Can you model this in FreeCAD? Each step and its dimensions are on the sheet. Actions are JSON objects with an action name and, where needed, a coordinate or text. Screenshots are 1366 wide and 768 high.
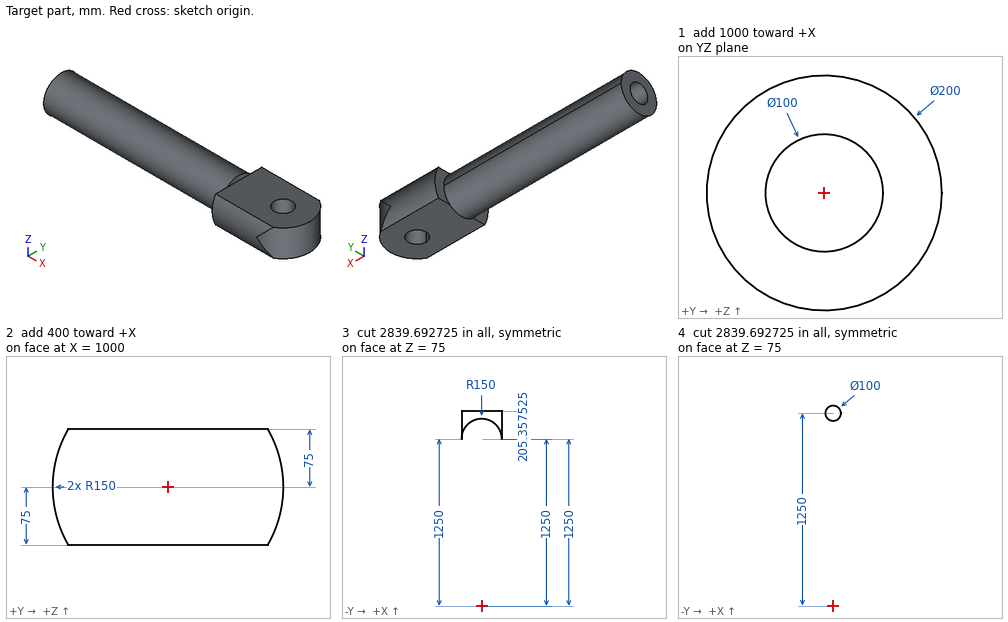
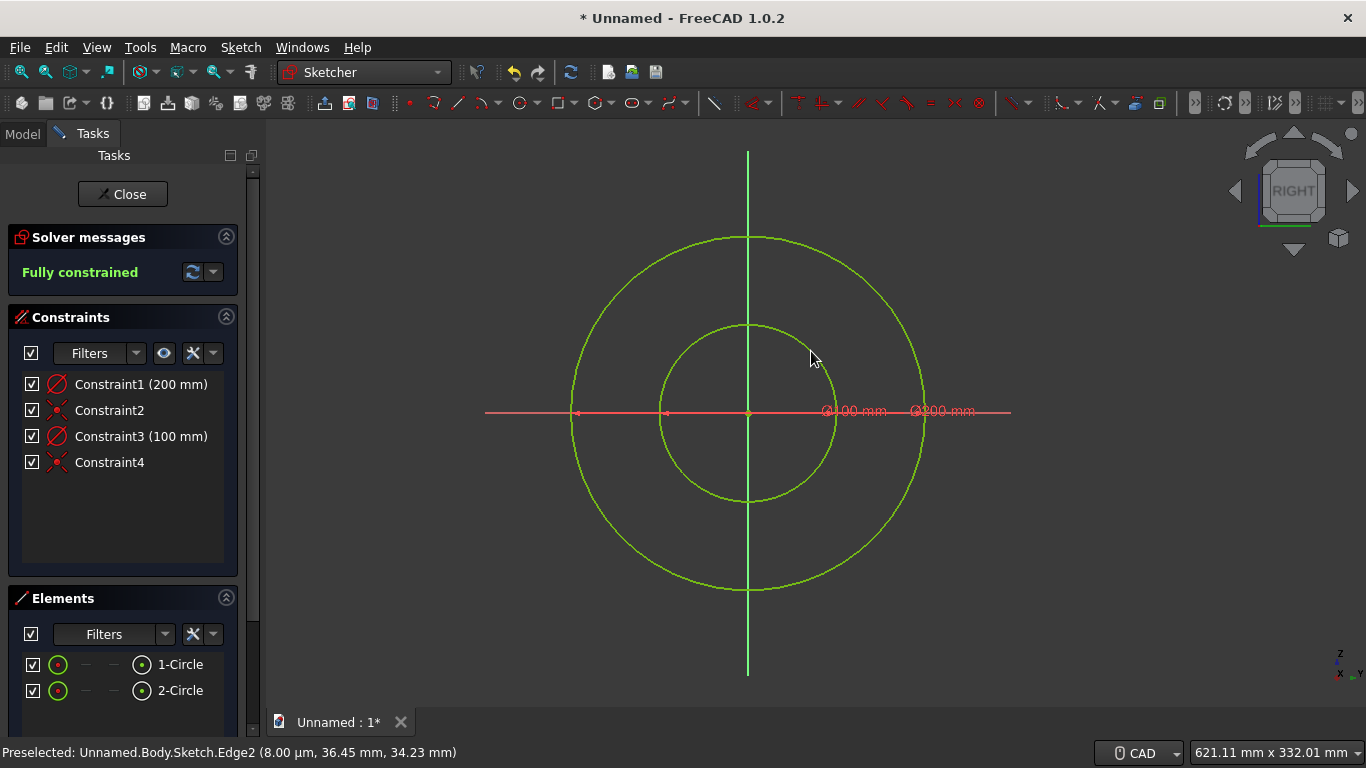
{"action": "left_click", "coordinate": [123, 194]}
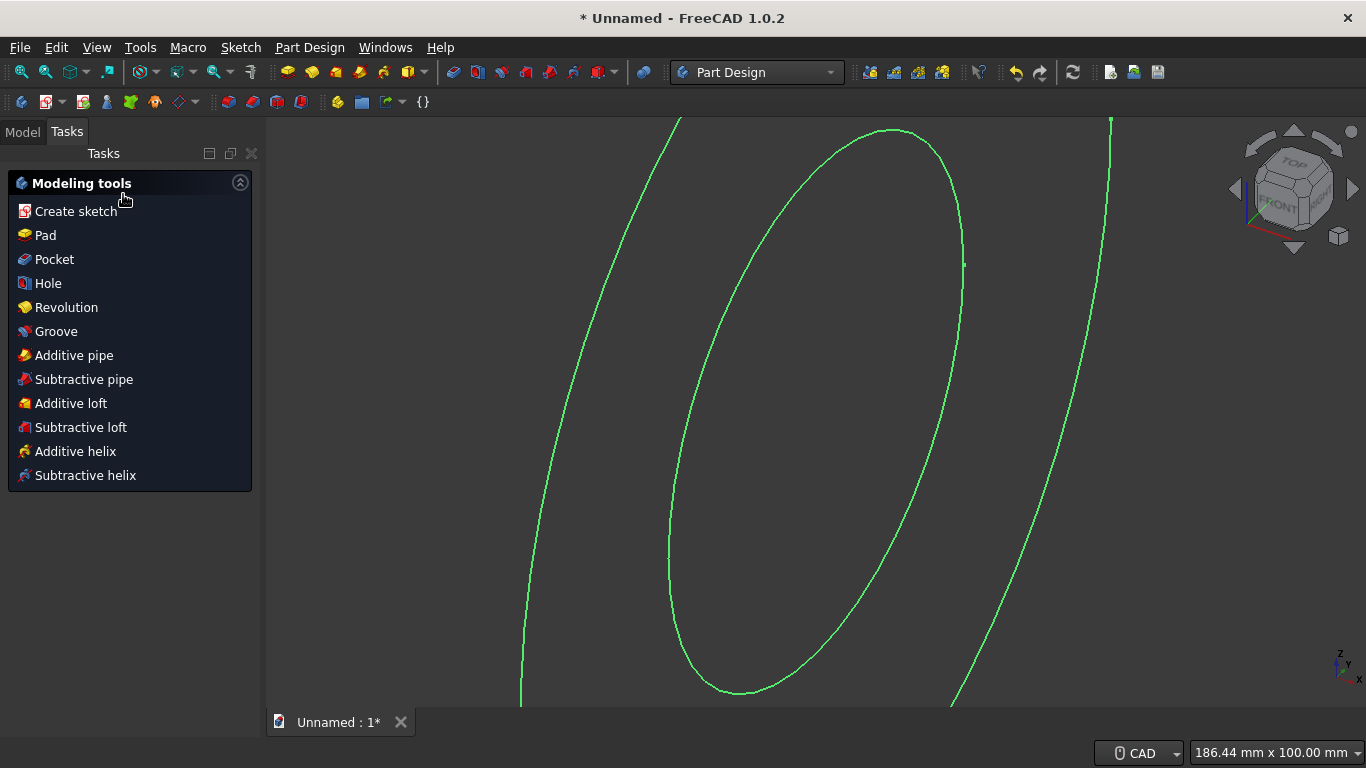
{"action": "left_click", "coordinate": [288, 72]}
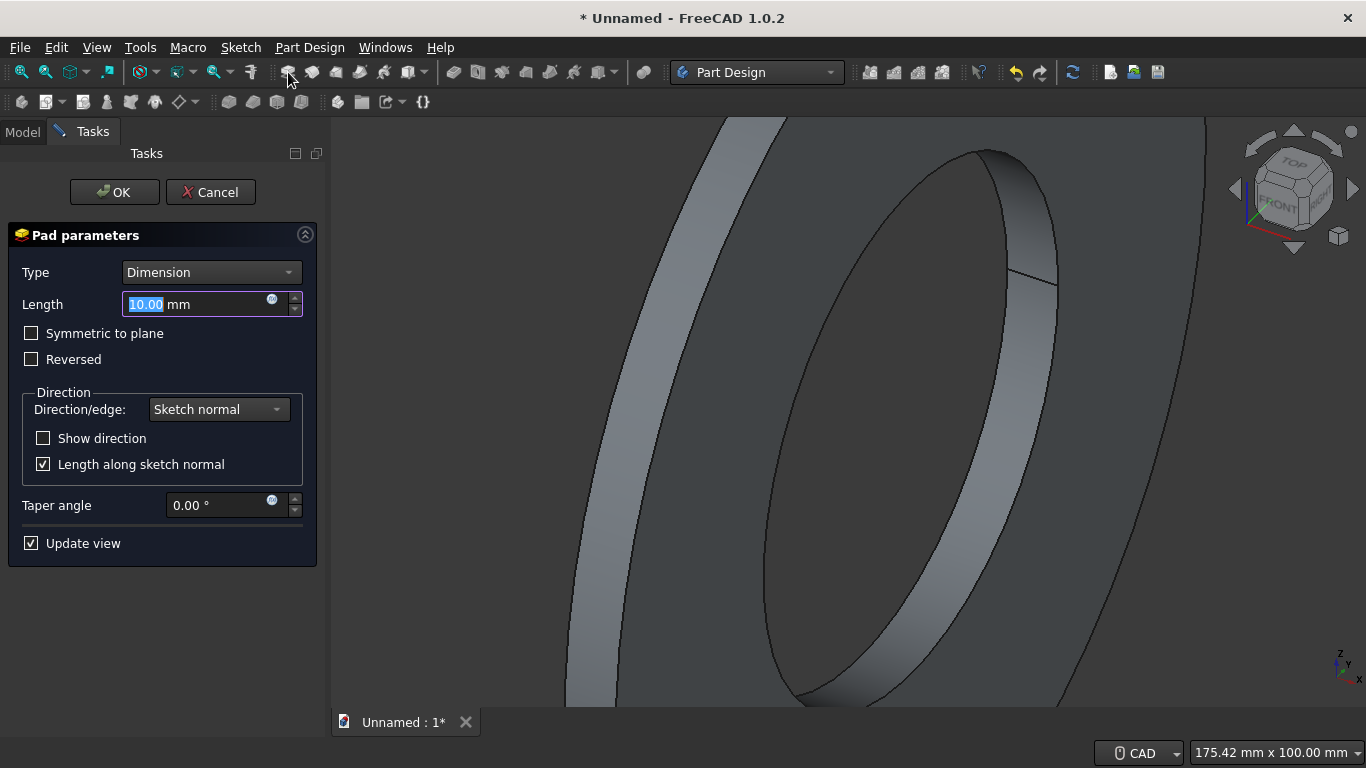
{"action": "type", "text": "1000"}
{"action": "key", "text": "Tab"}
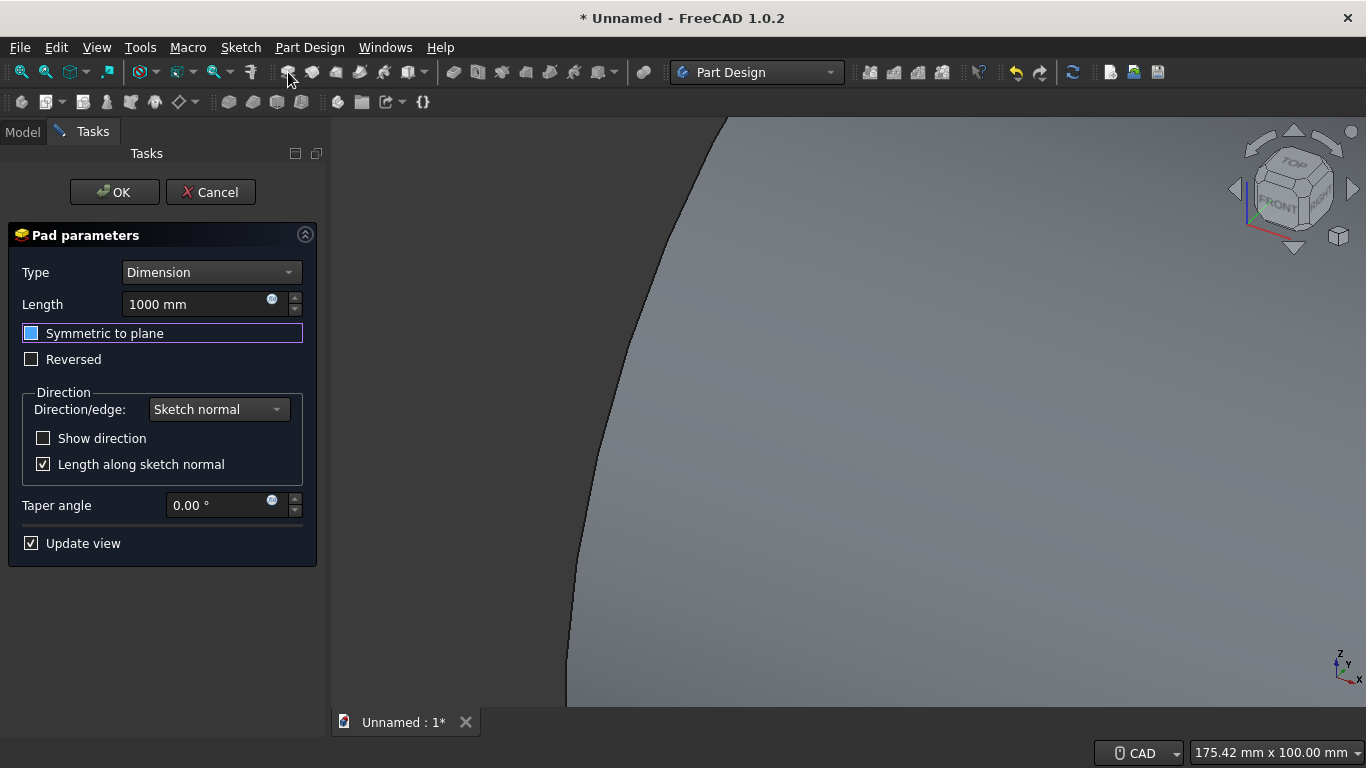
{"action": "left_click", "coordinate": [115, 192]}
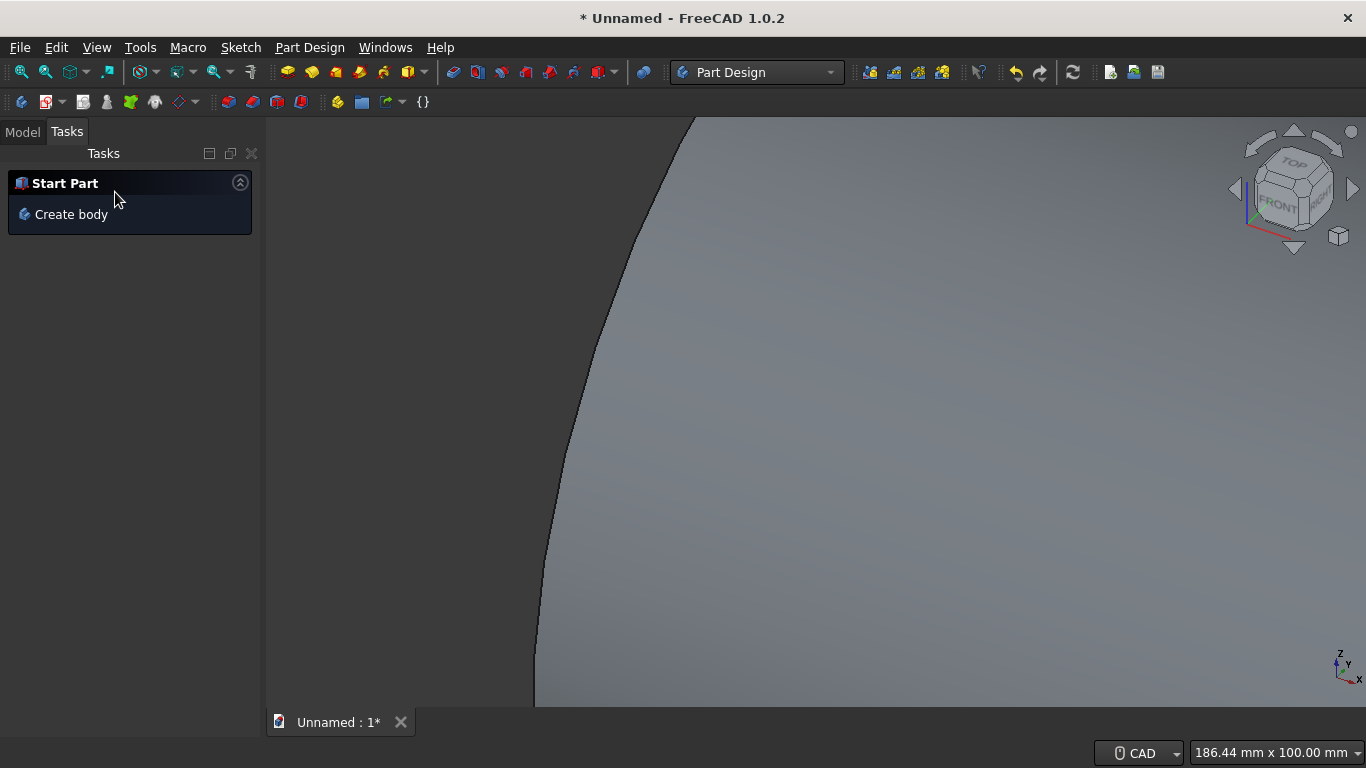
{"action": "left_click", "coordinate": [22, 72]}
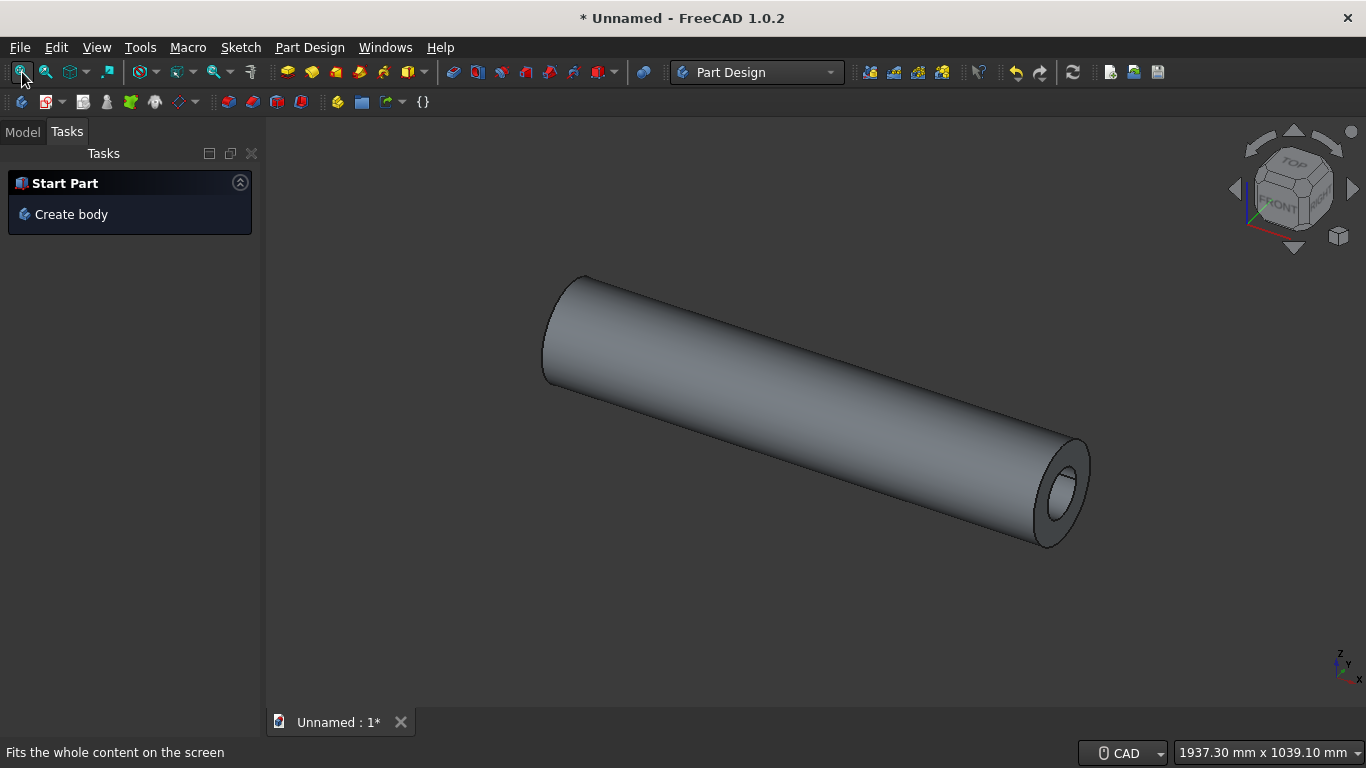
{"action": "left_click", "coordinate": [1046, 535]}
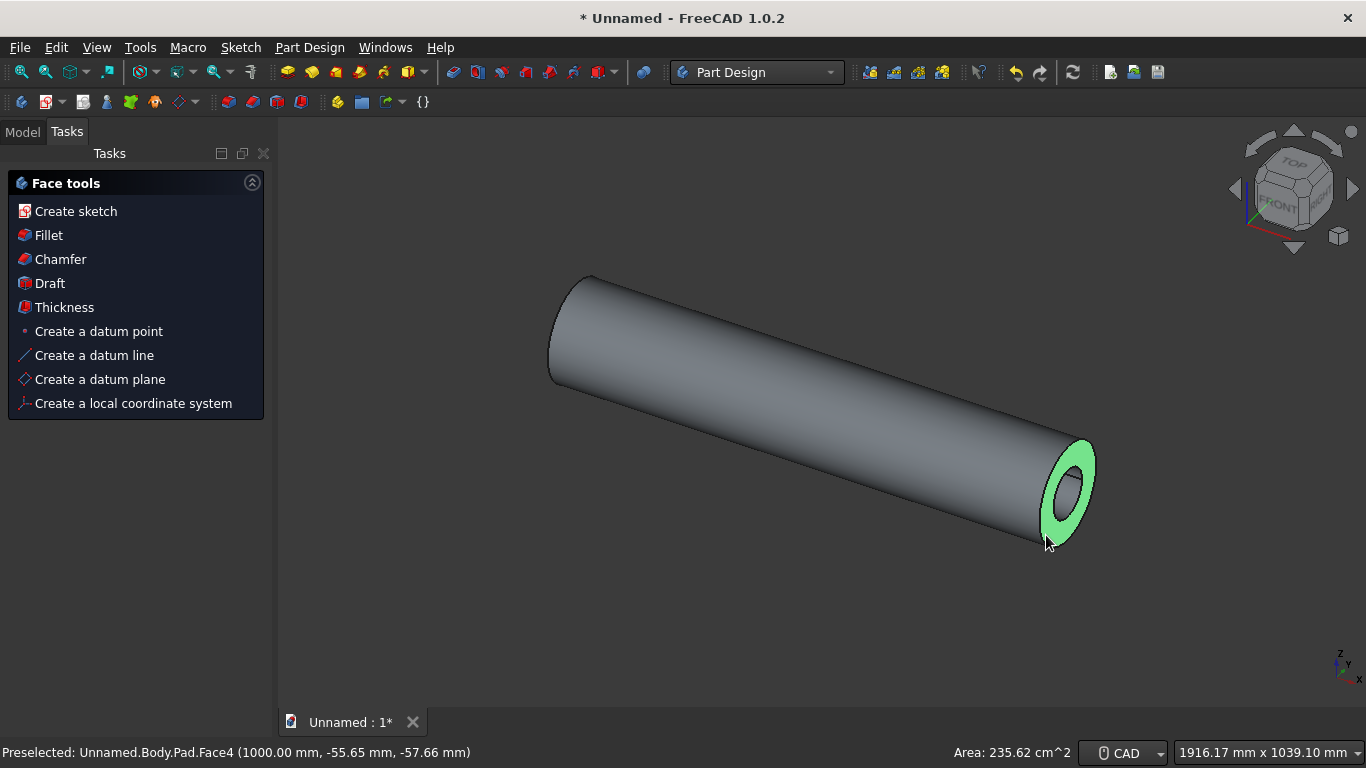
{"action": "left_click", "coordinate": [46, 102]}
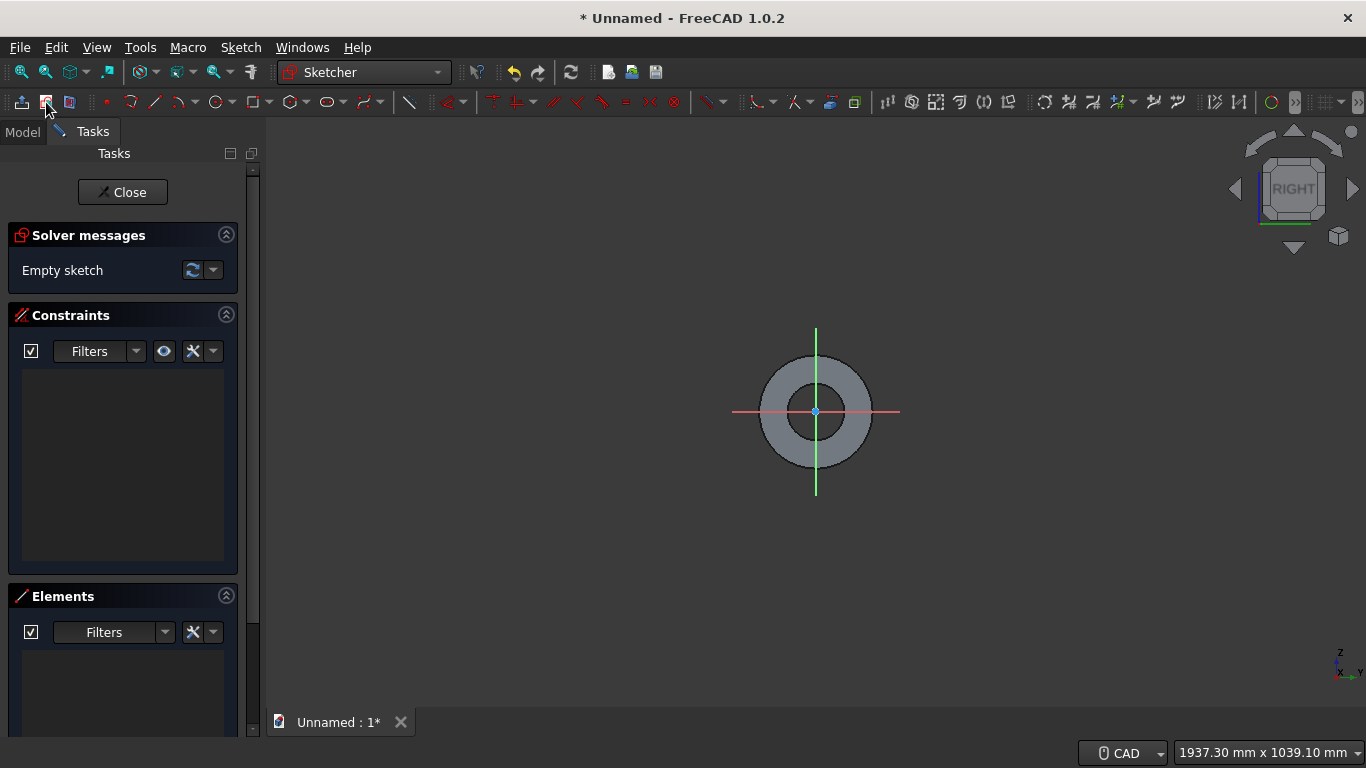
{"action": "scroll", "coordinate": [838, 412], "scroll_direction": "up", "scroll_amount": 7}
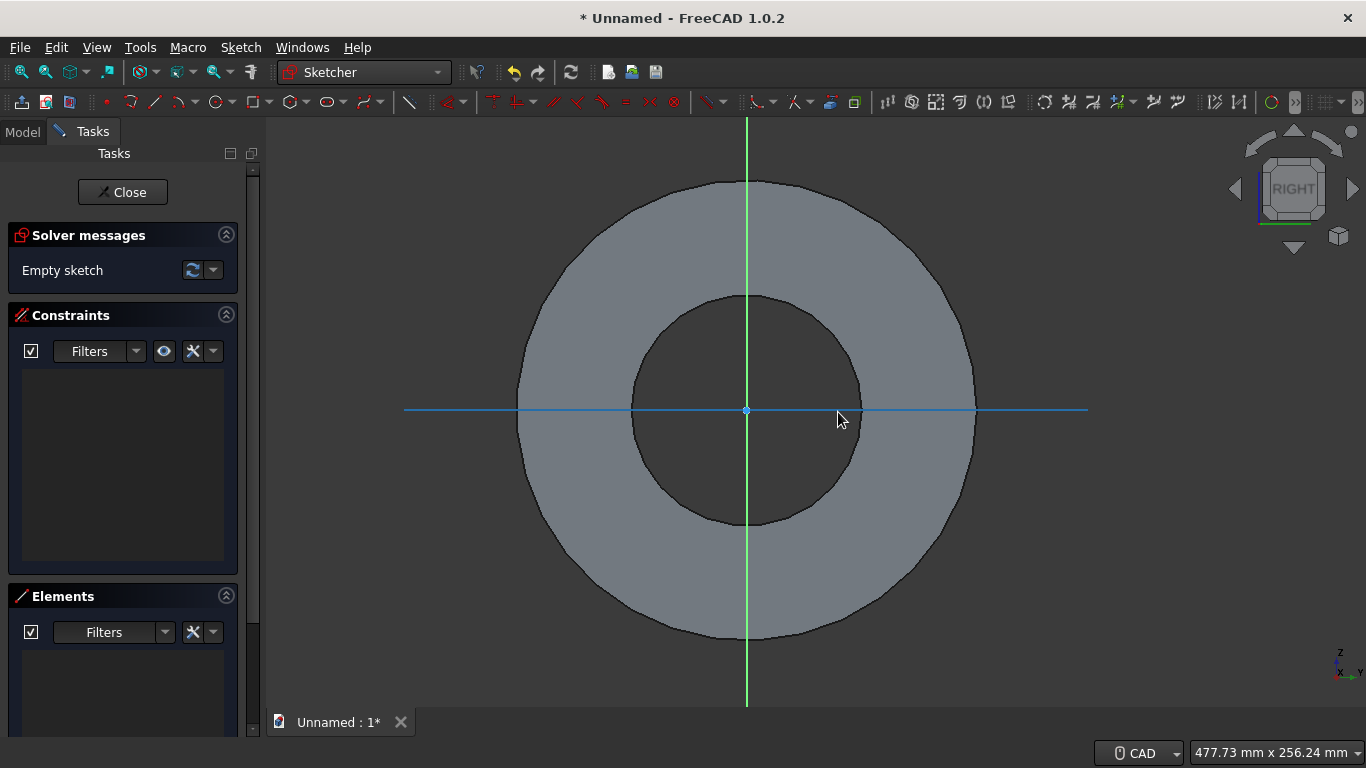
{"action": "left_click", "coordinate": [156, 102]}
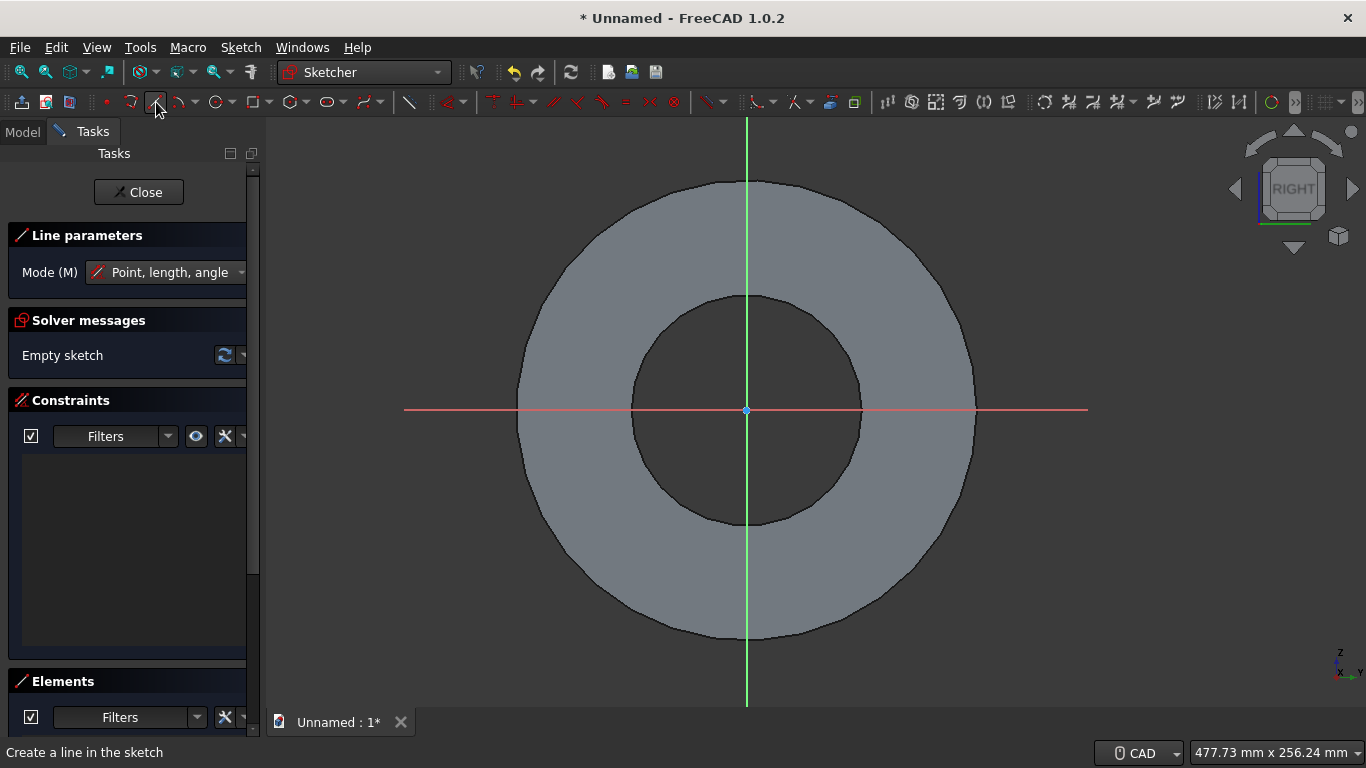
{"action": "left_click", "coordinate": [1046, 238]}
{"action": "left_click", "coordinate": [448, 238]}